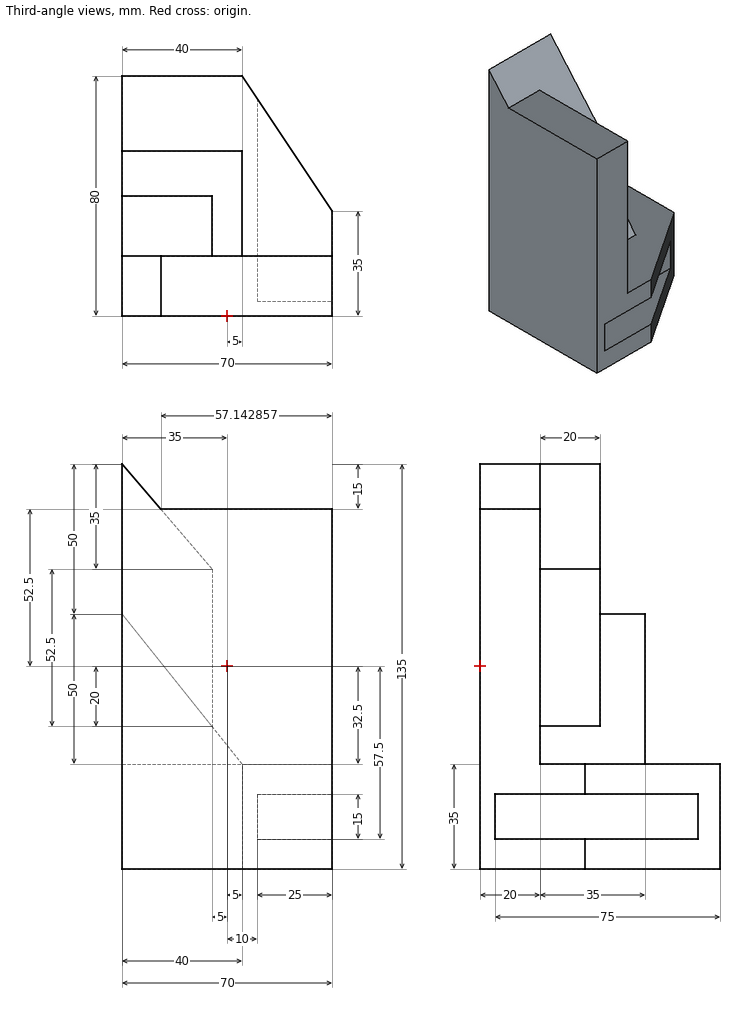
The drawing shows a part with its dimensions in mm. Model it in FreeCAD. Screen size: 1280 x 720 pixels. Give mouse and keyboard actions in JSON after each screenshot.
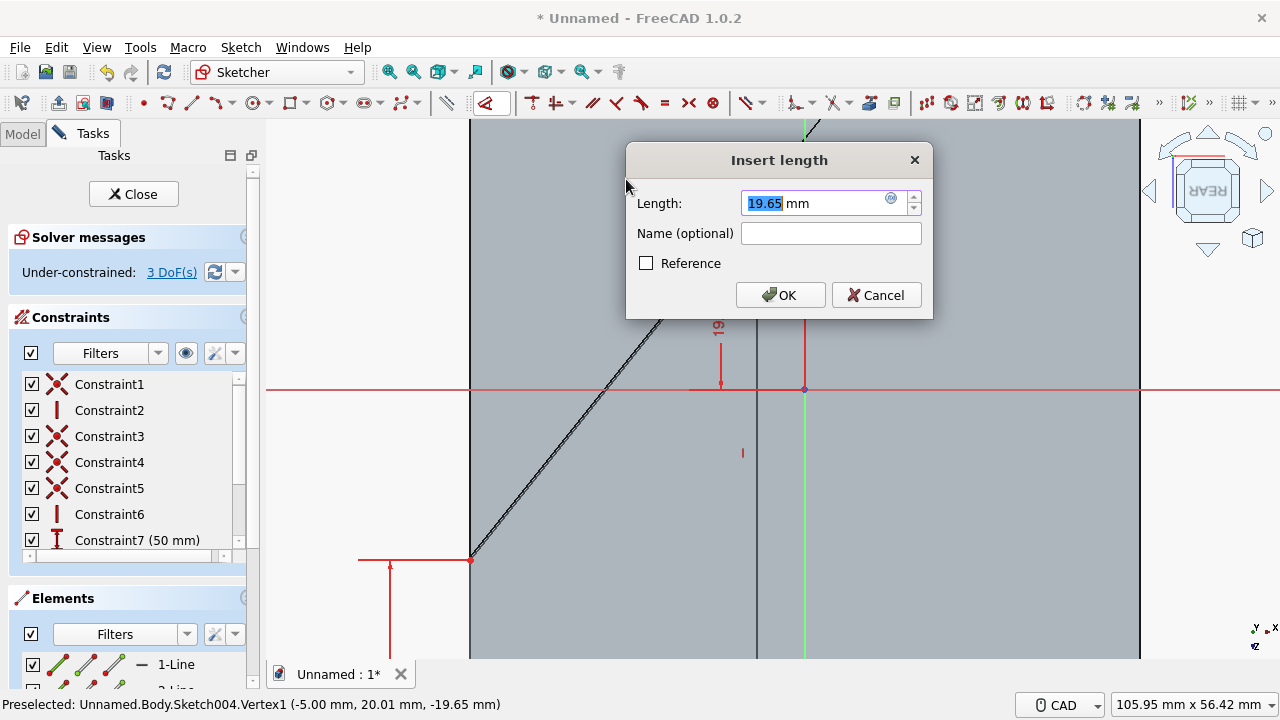
{"action": "type", "text": "20"}
{"action": "key", "text": "Return"}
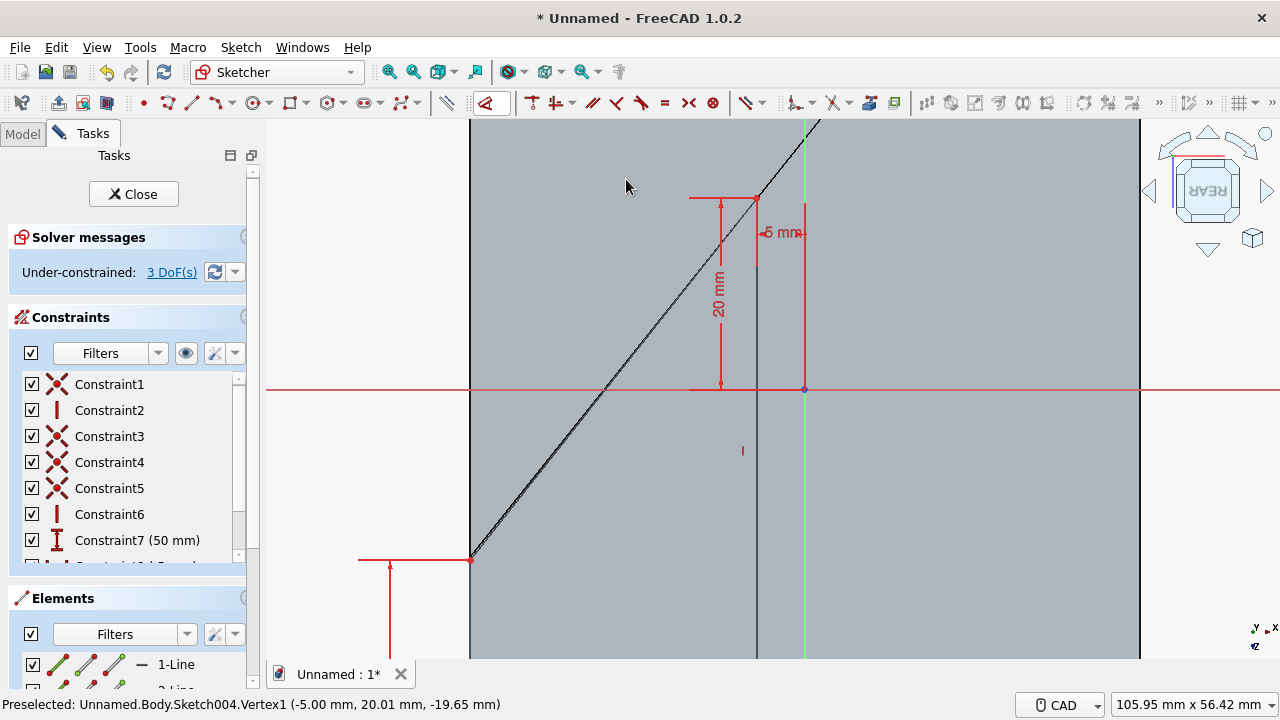
{"action": "left_click", "coordinate": [470, 560]}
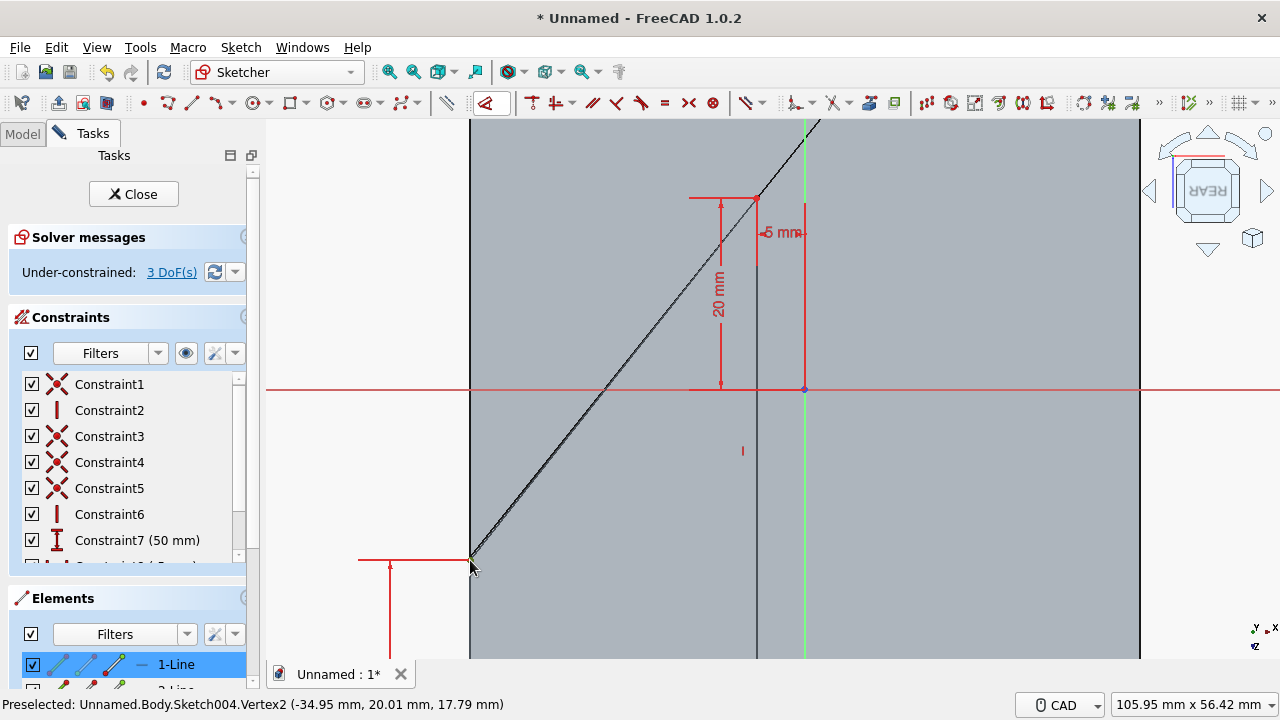
{"action": "left_click", "coordinate": [504, 104]}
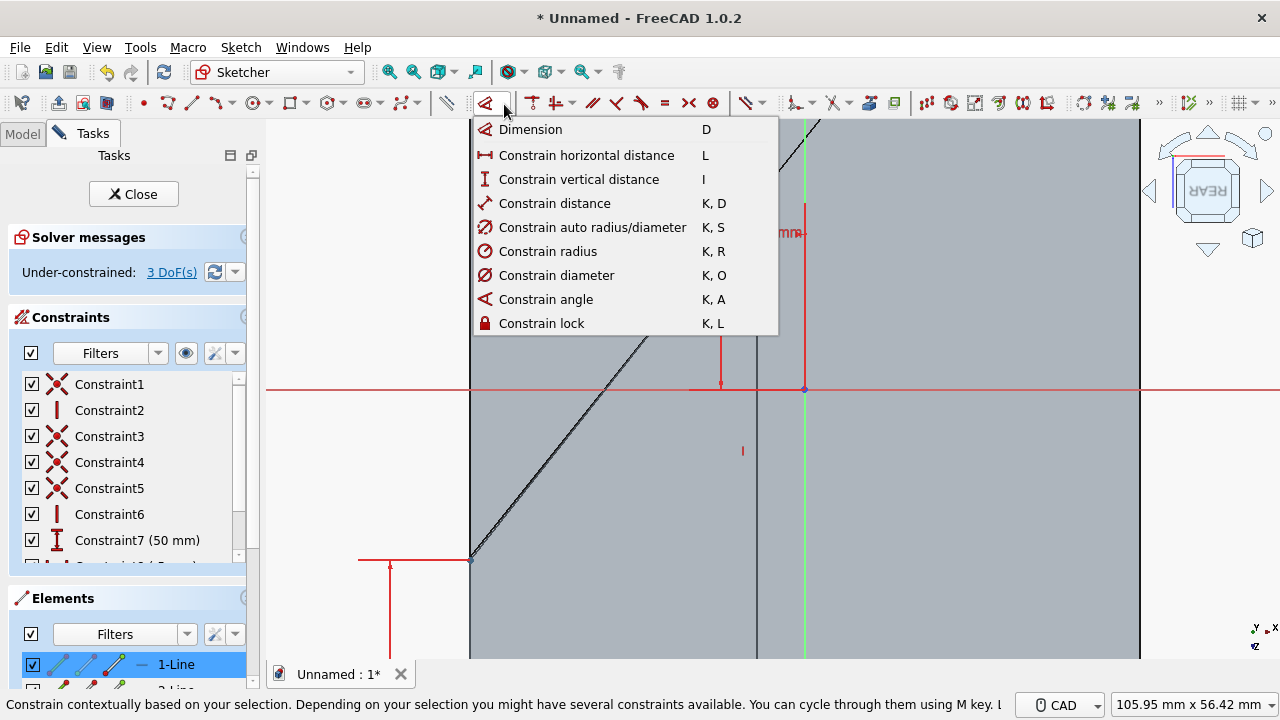
{"action": "left_click", "coordinate": [626, 155]}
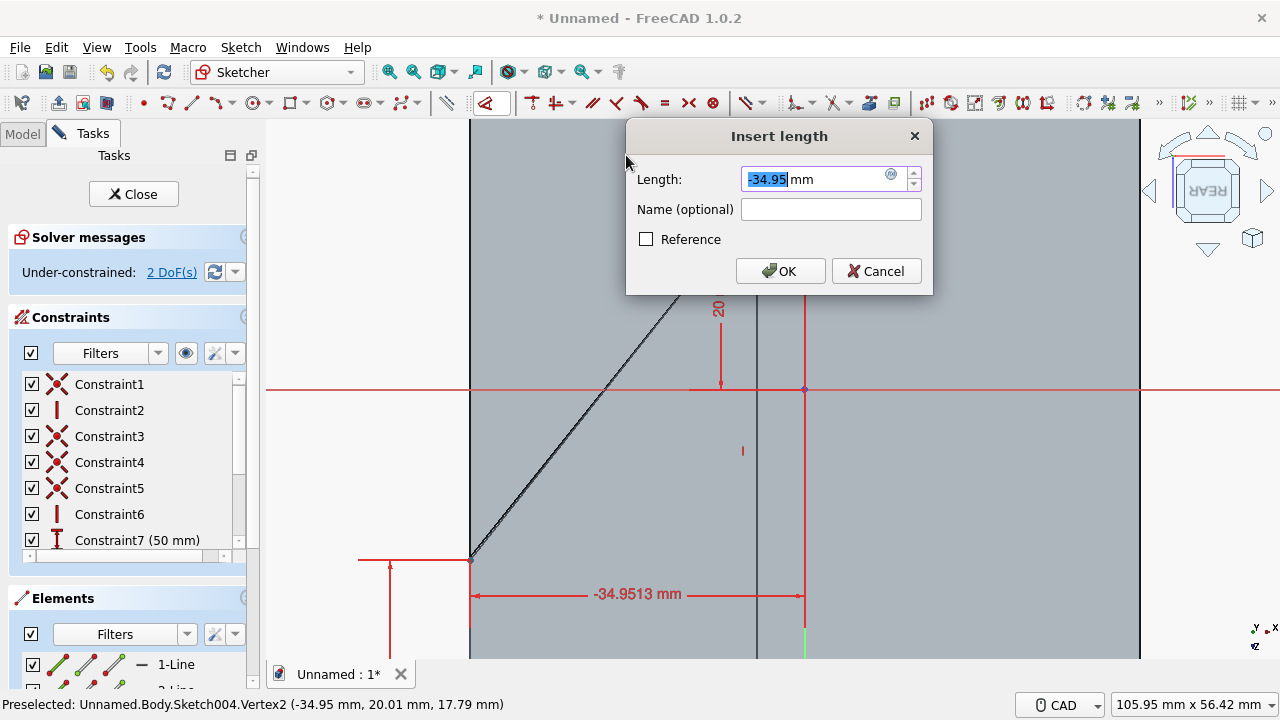
{"action": "type", "text": "-35"}
{"action": "key", "text": "Return"}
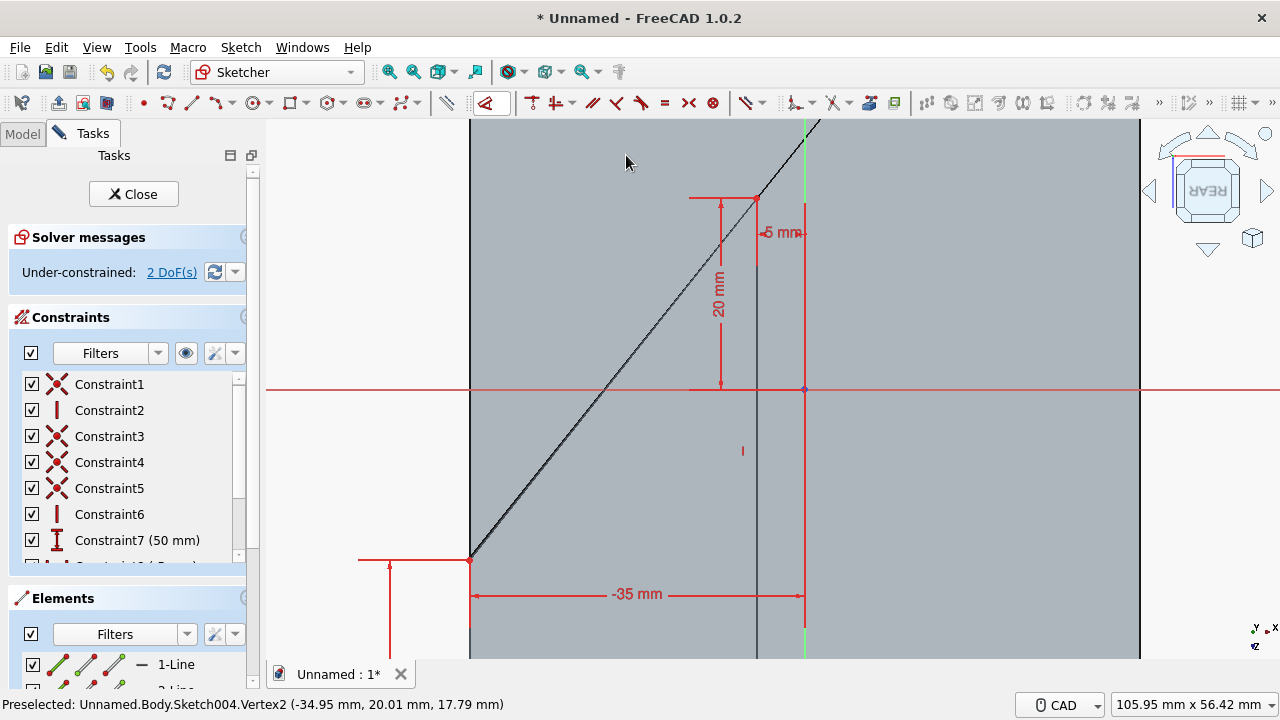
{"action": "scroll", "coordinate": [759, 203], "scroll_direction": "down", "scroll_amount": 4}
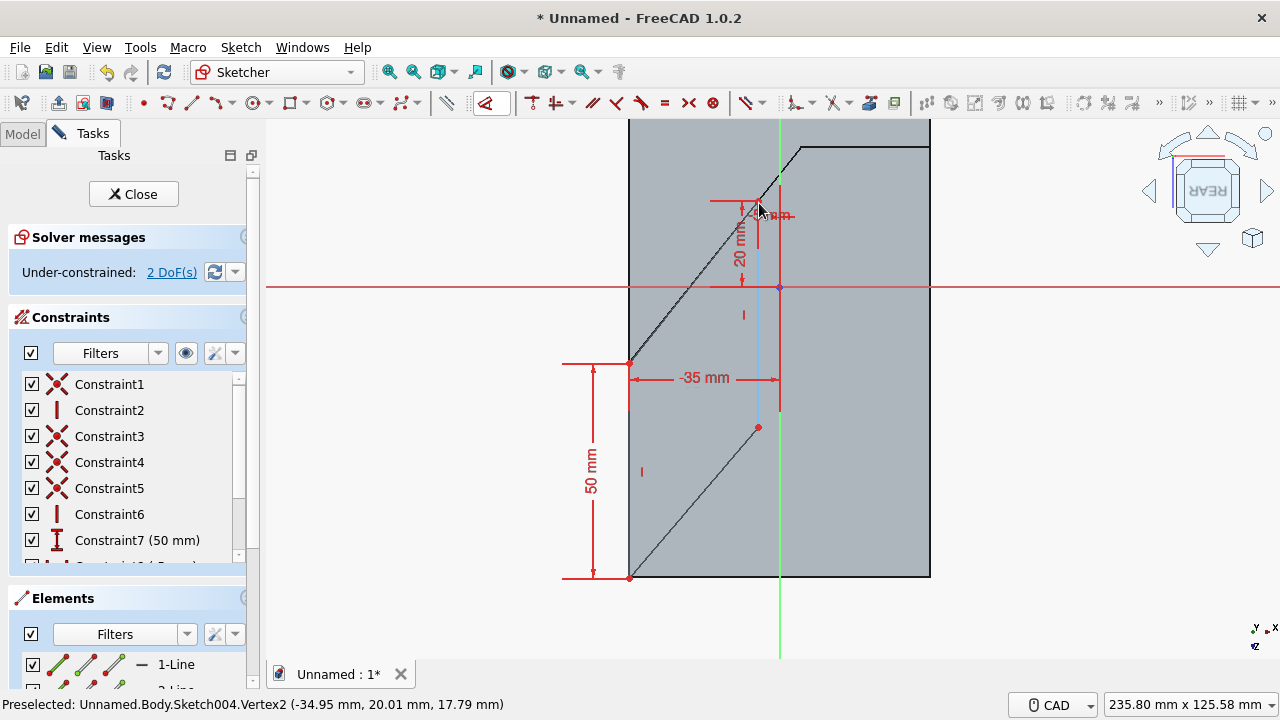
{"action": "left_click", "coordinate": [668, 533]}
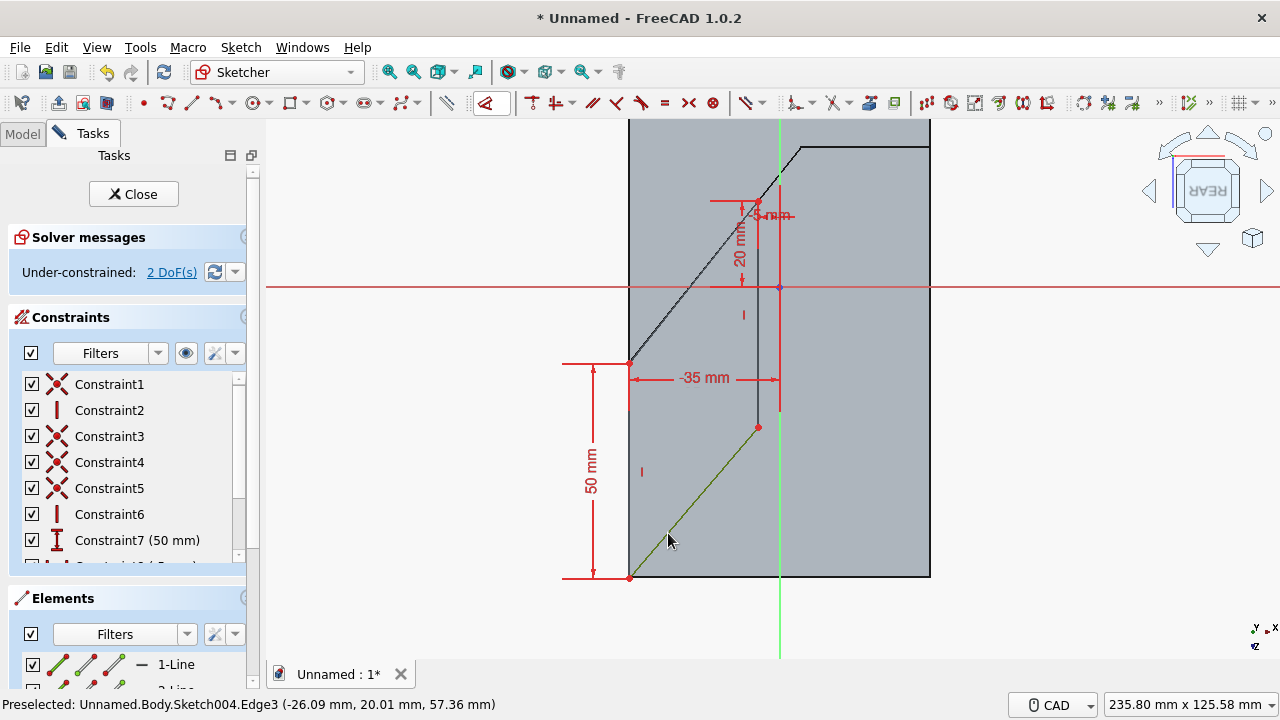
{"action": "key", "text": "i"}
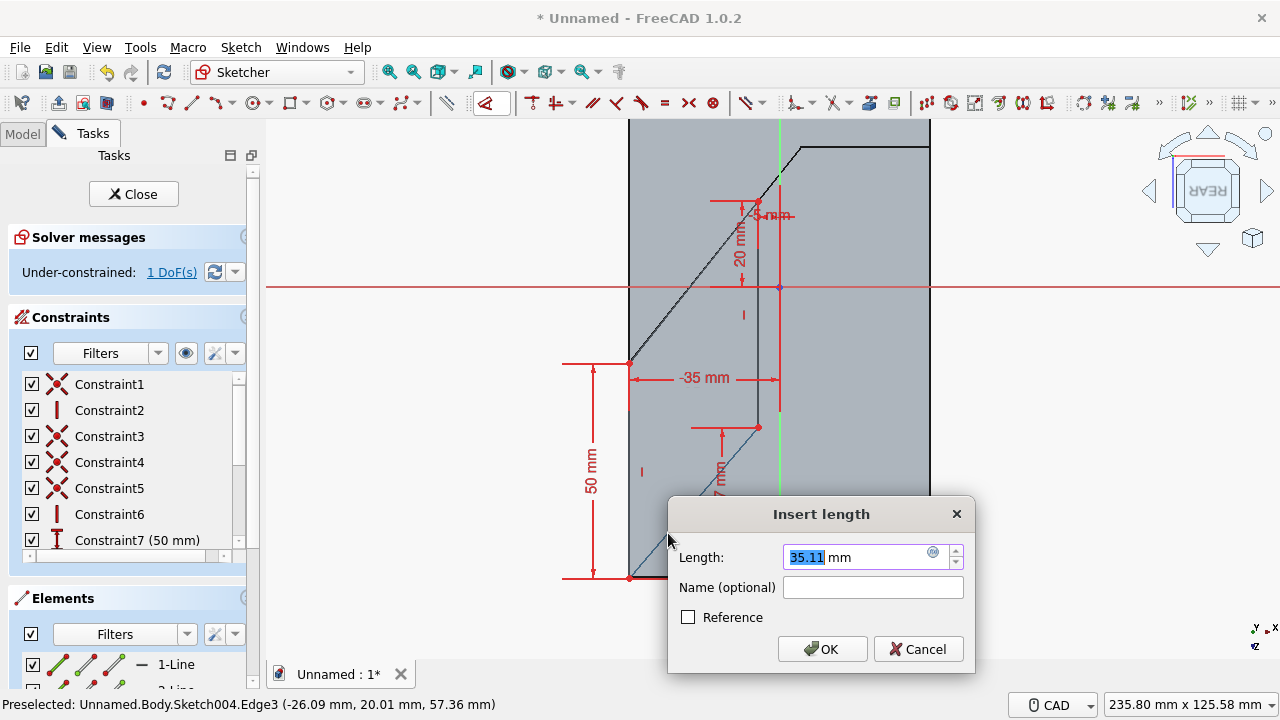
{"action": "type", "text": "35"}
{"action": "key", "text": "Return"}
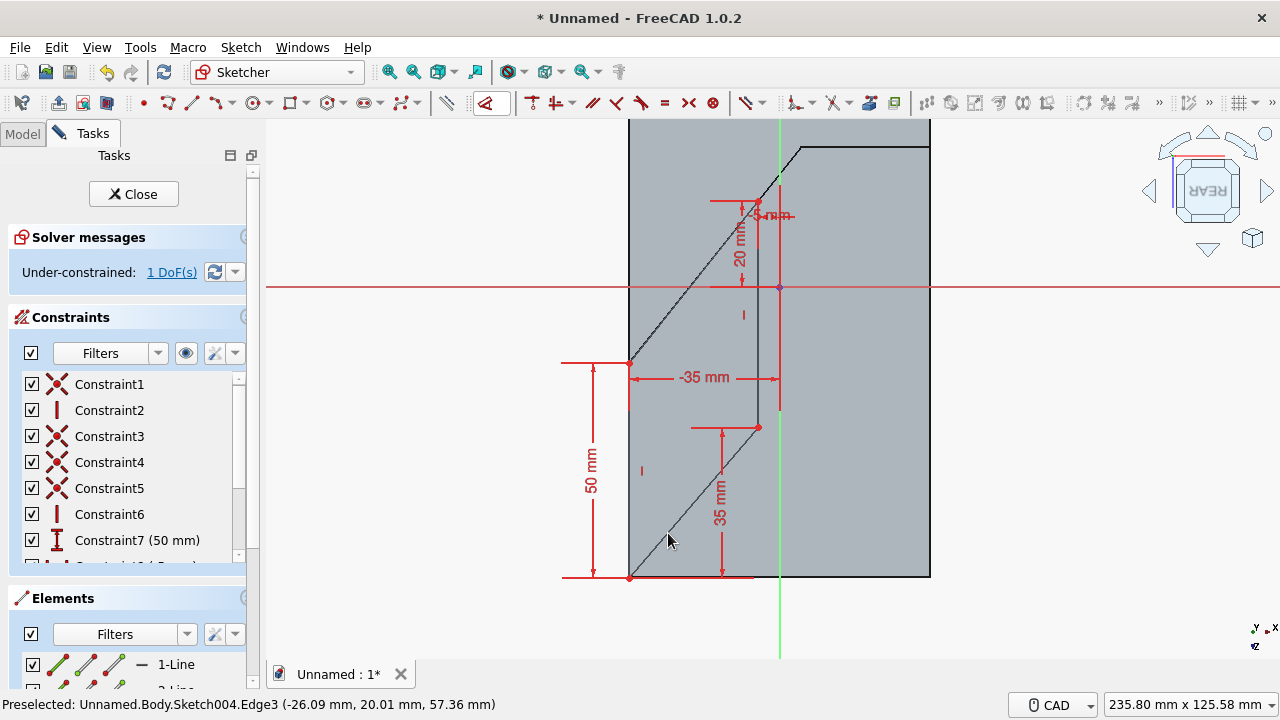
{"action": "left_click", "coordinate": [758, 360]}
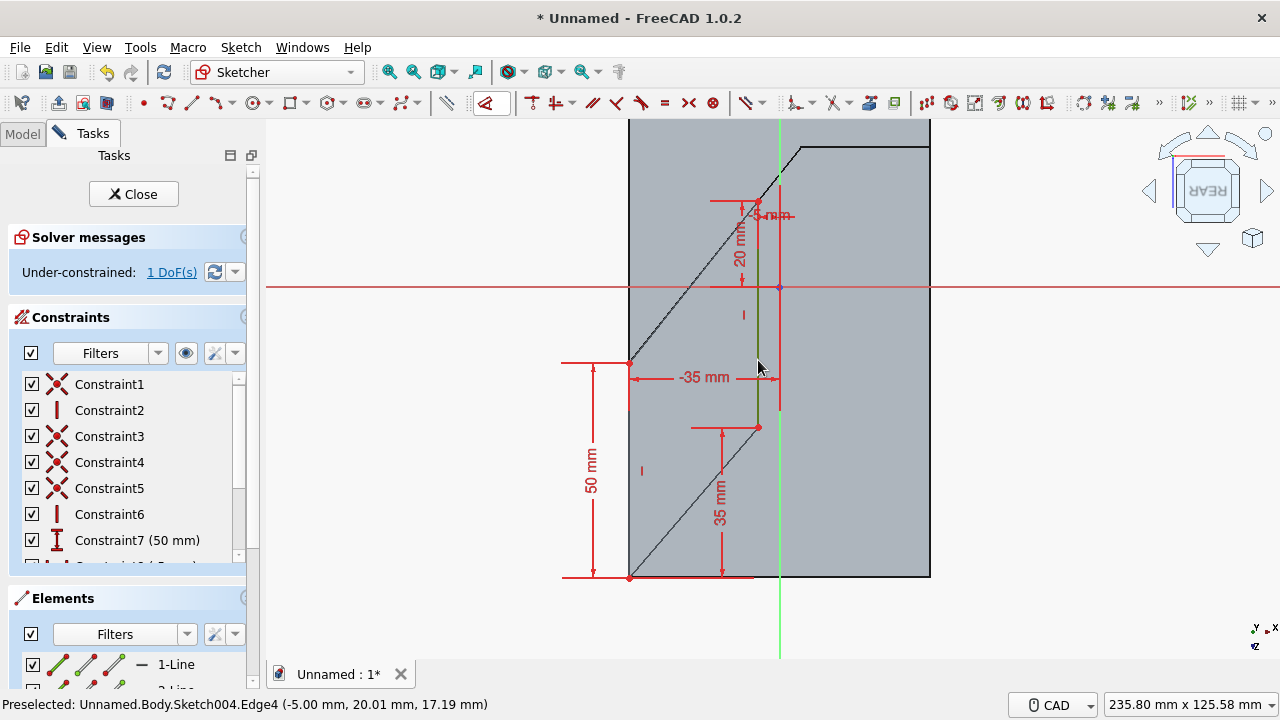
{"action": "key", "text": "i"}